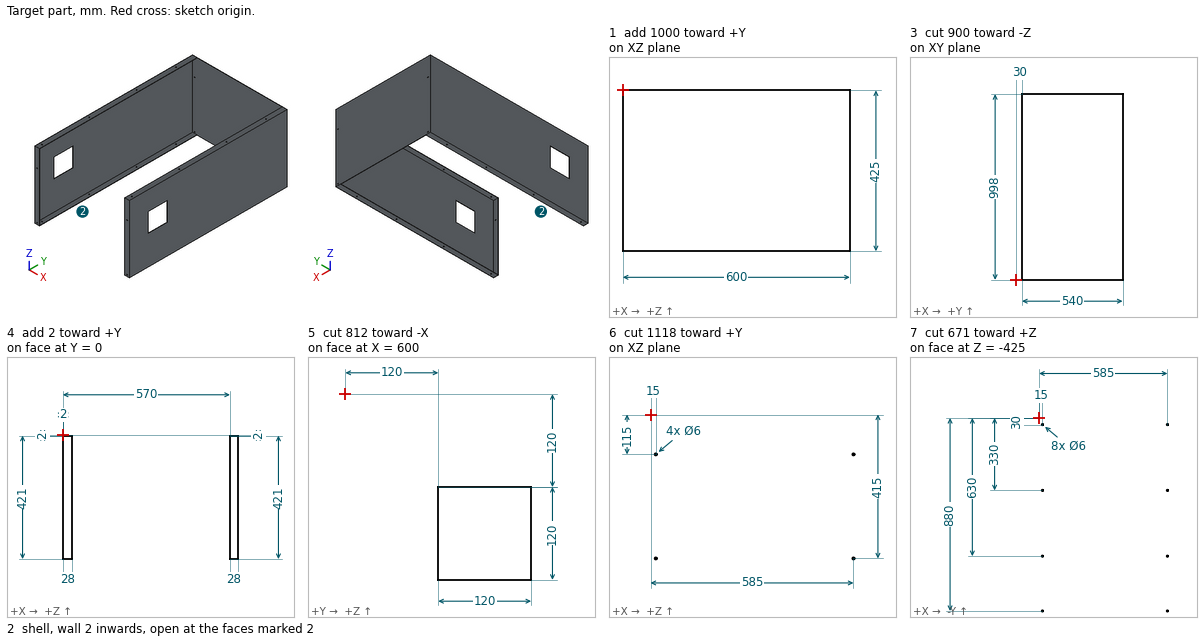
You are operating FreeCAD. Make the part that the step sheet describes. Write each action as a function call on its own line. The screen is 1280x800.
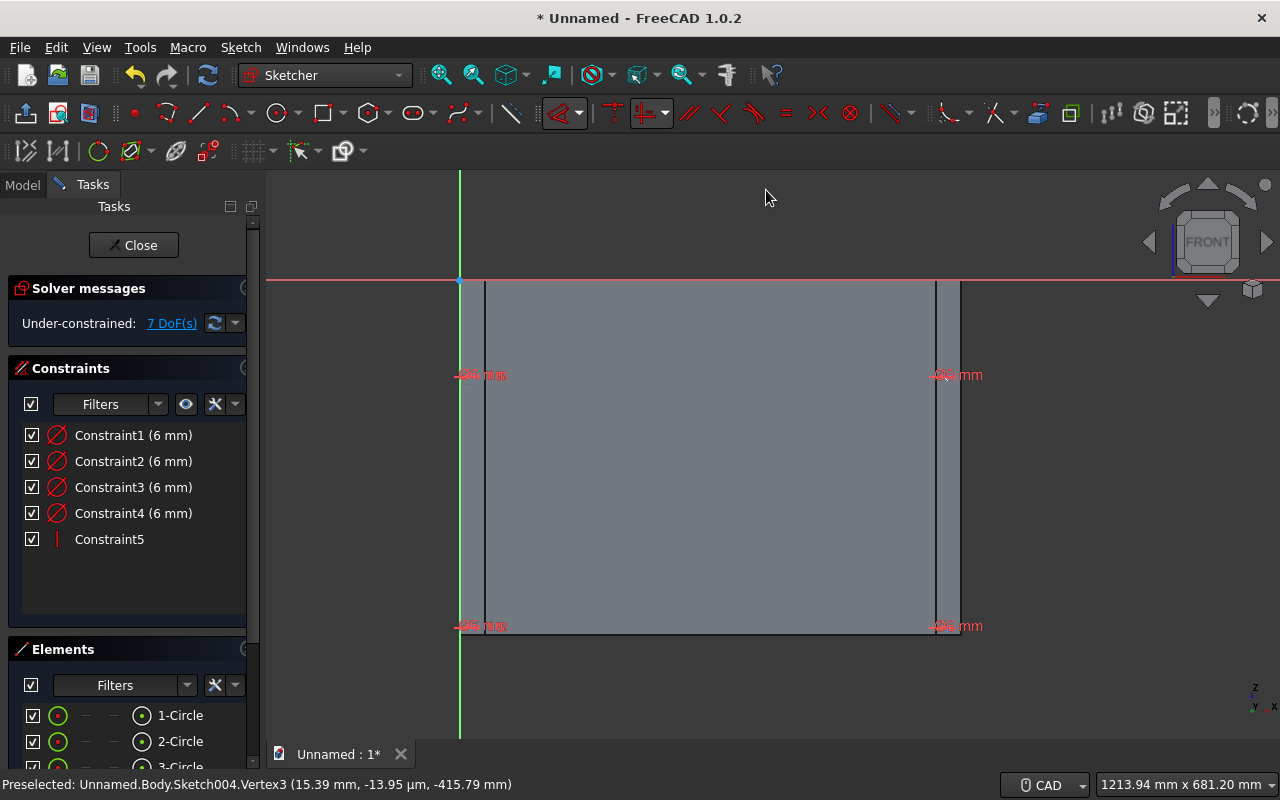
click(948, 628)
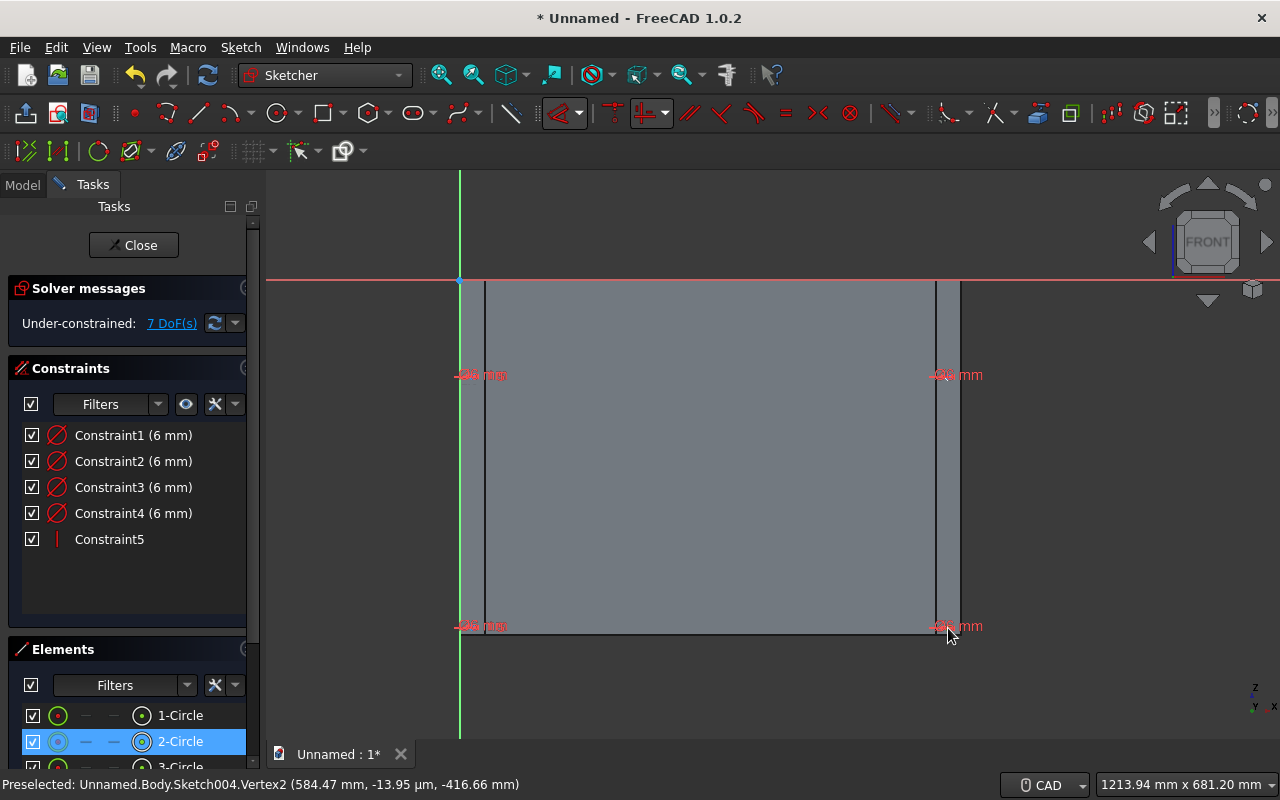
click(472, 628)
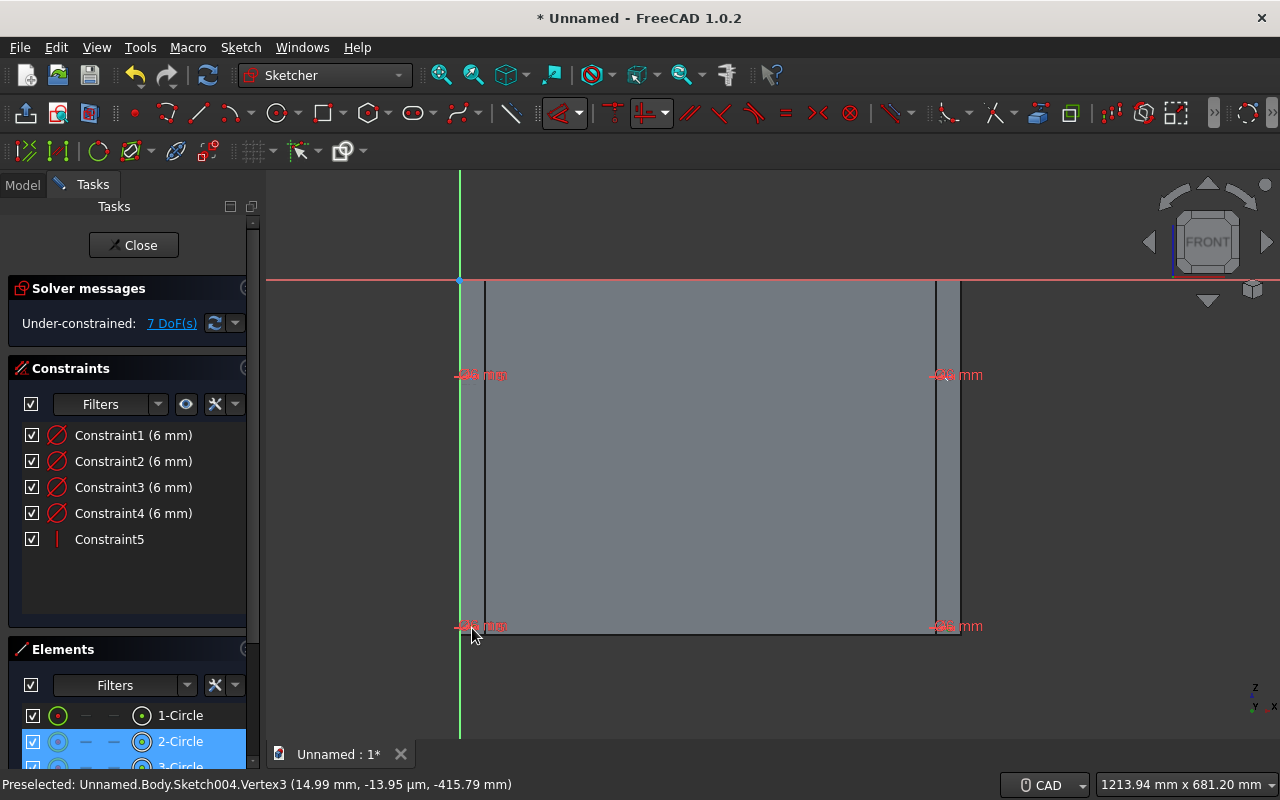
click(668, 114)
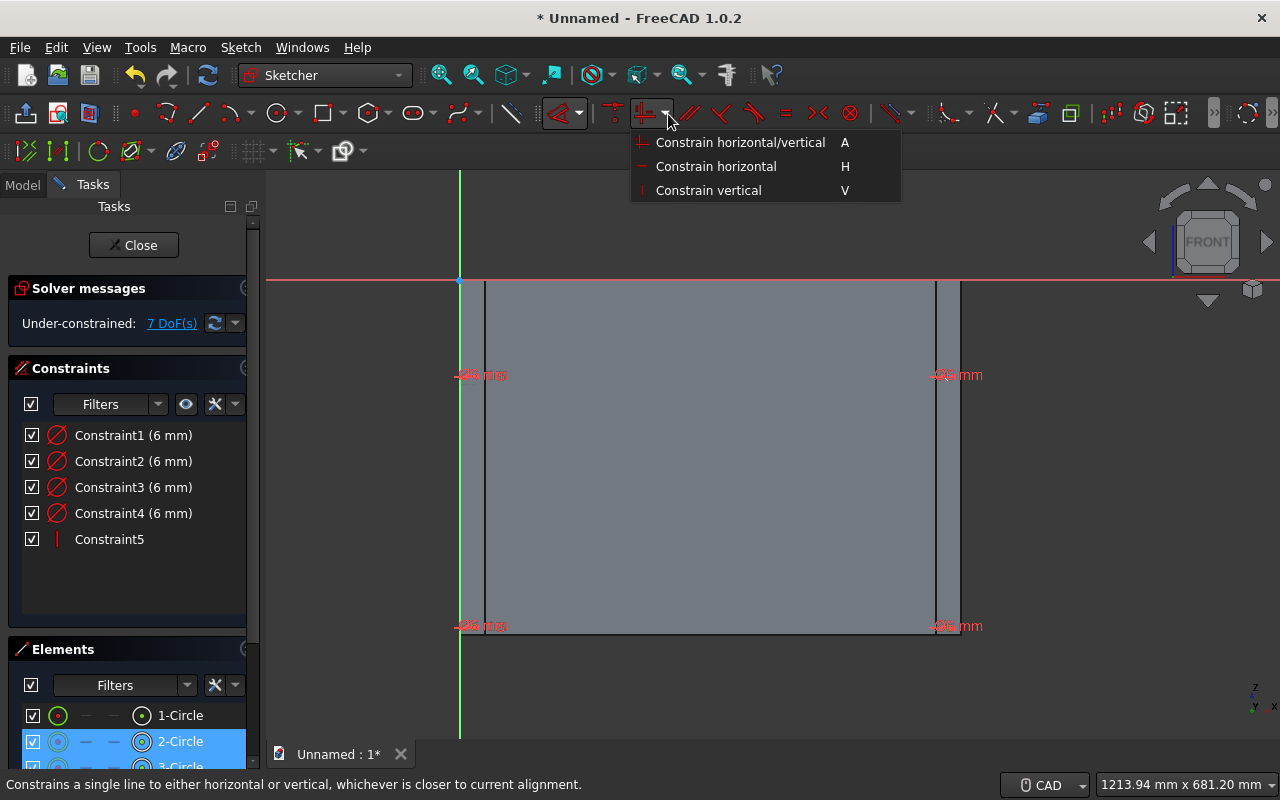
click(766, 166)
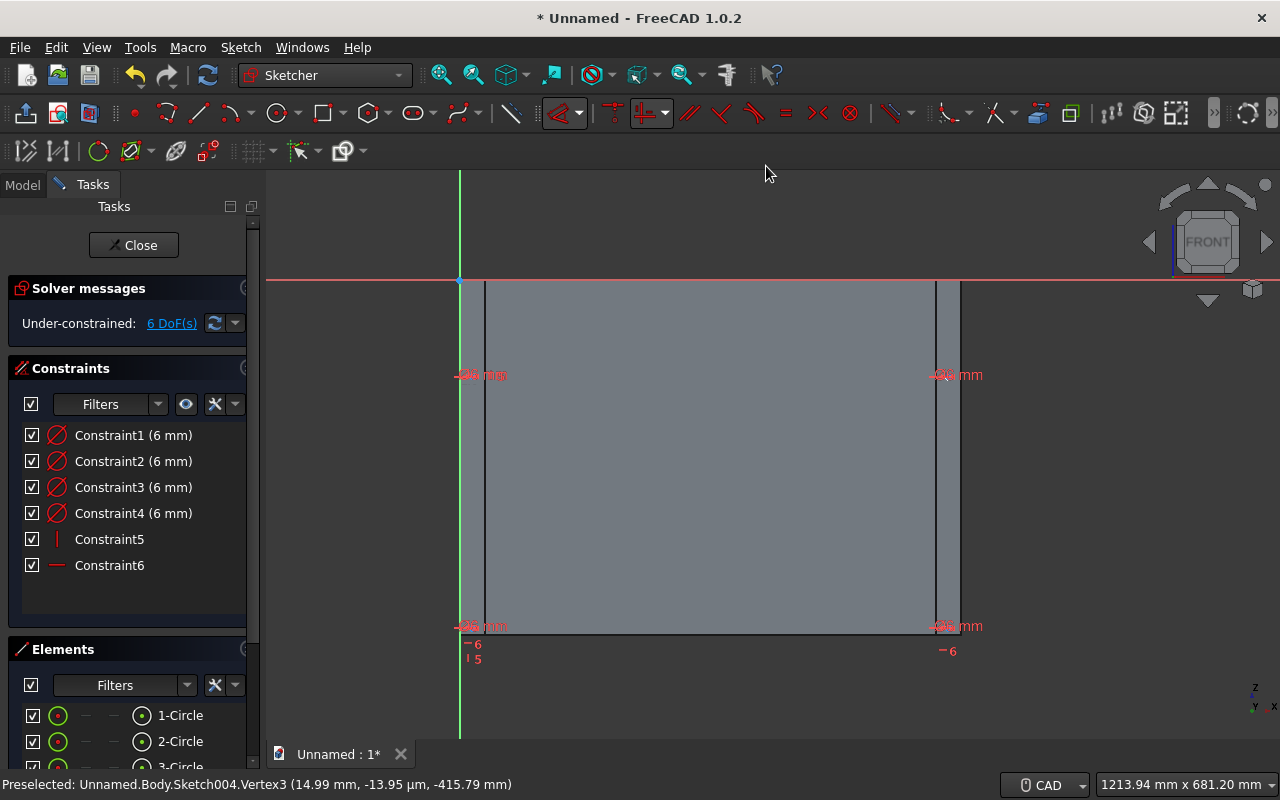
click(948, 628)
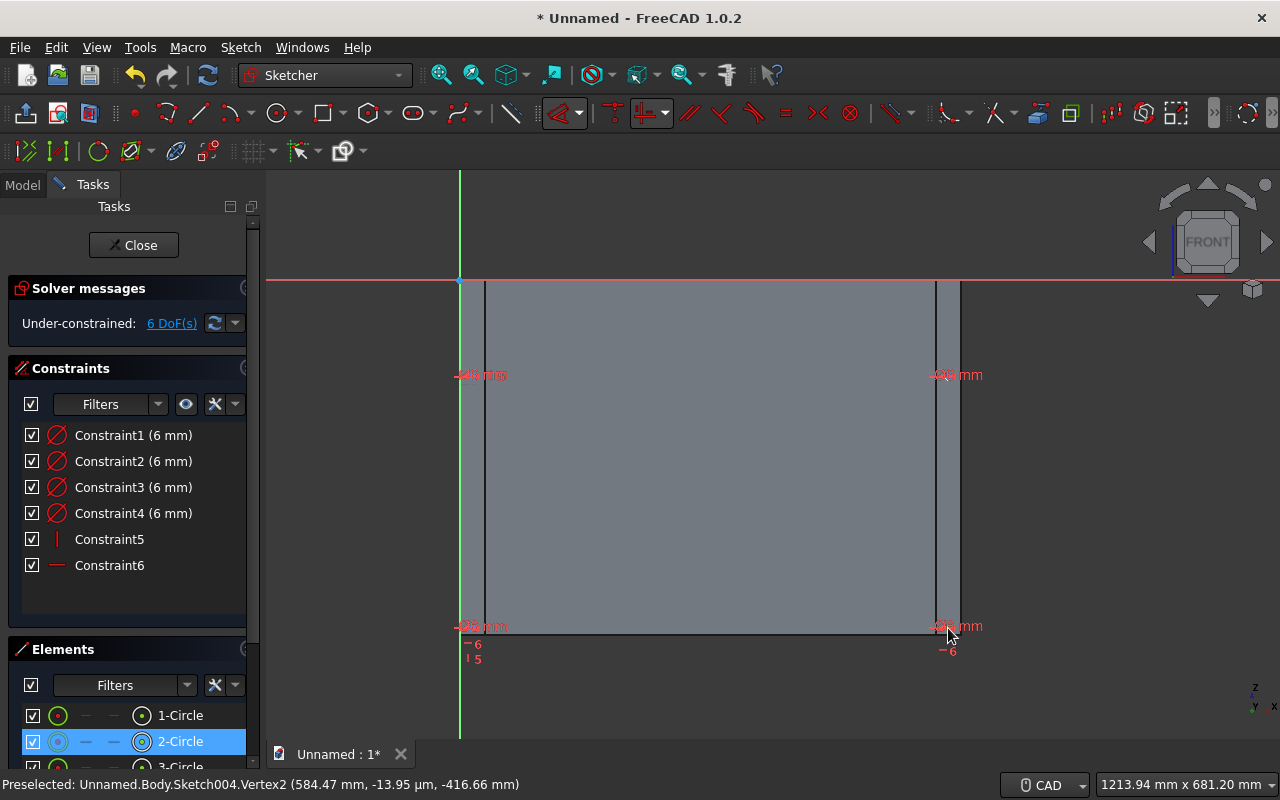
click(948, 377)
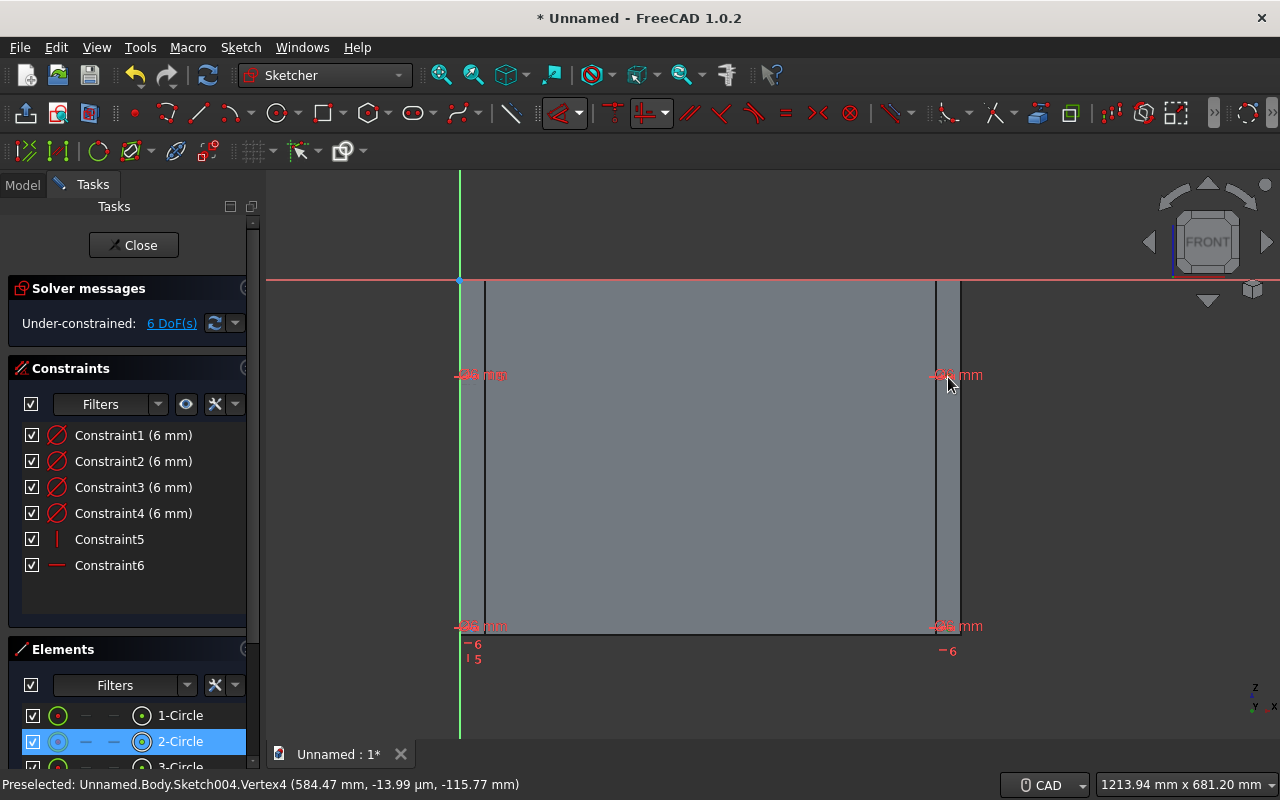
click(668, 114)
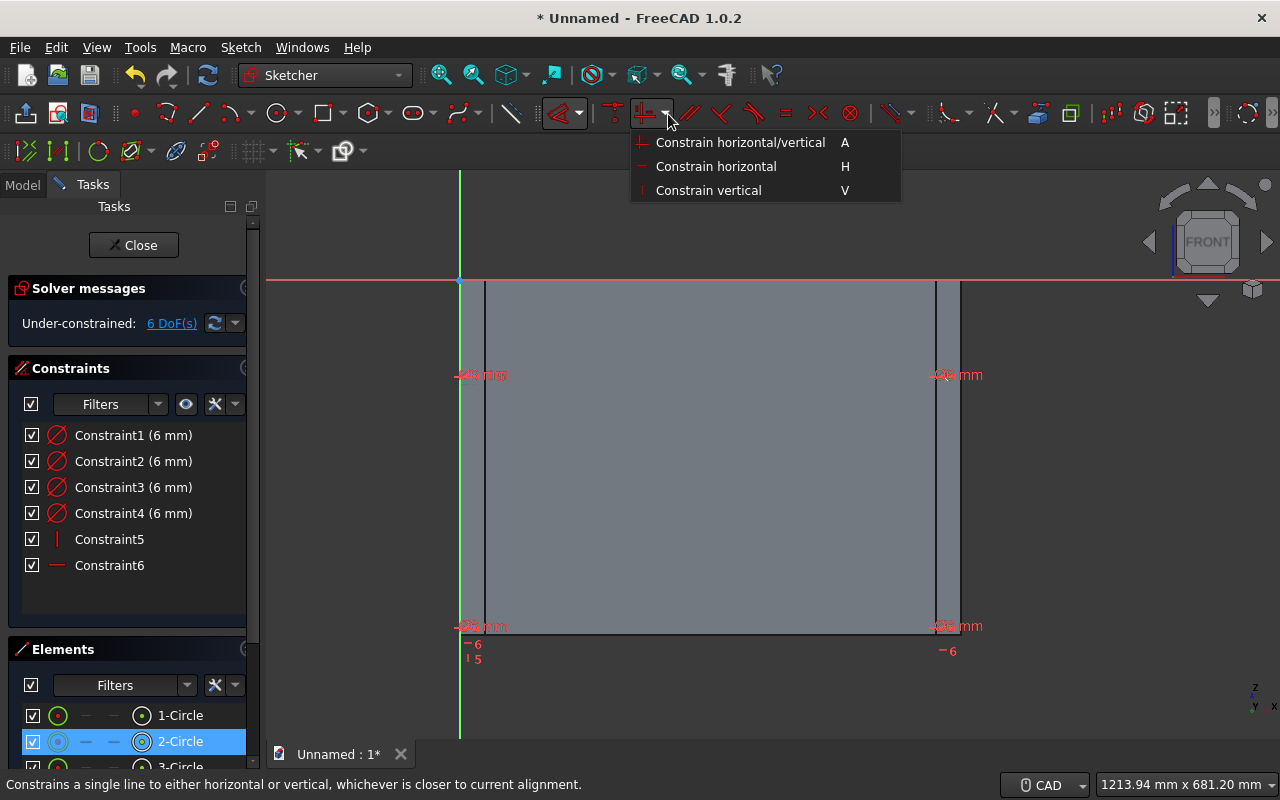
click(766, 190)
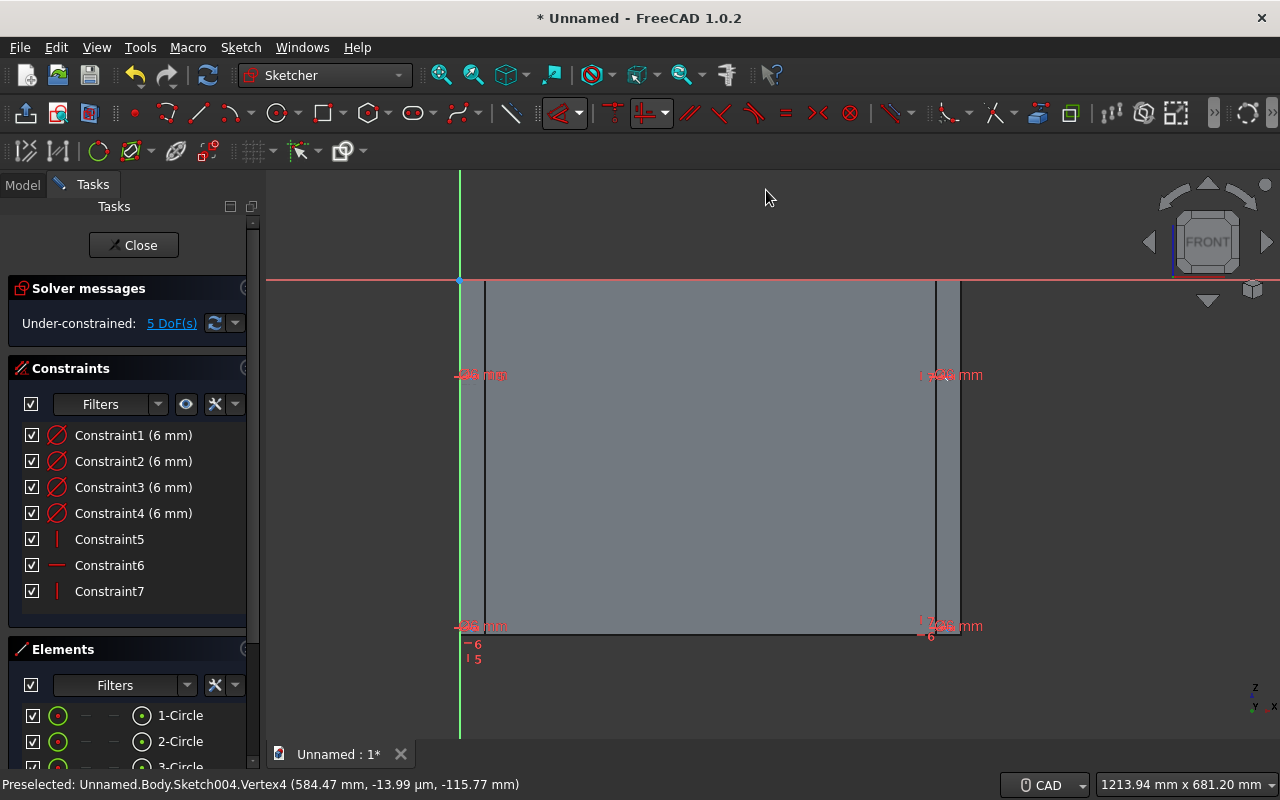
click(472, 377)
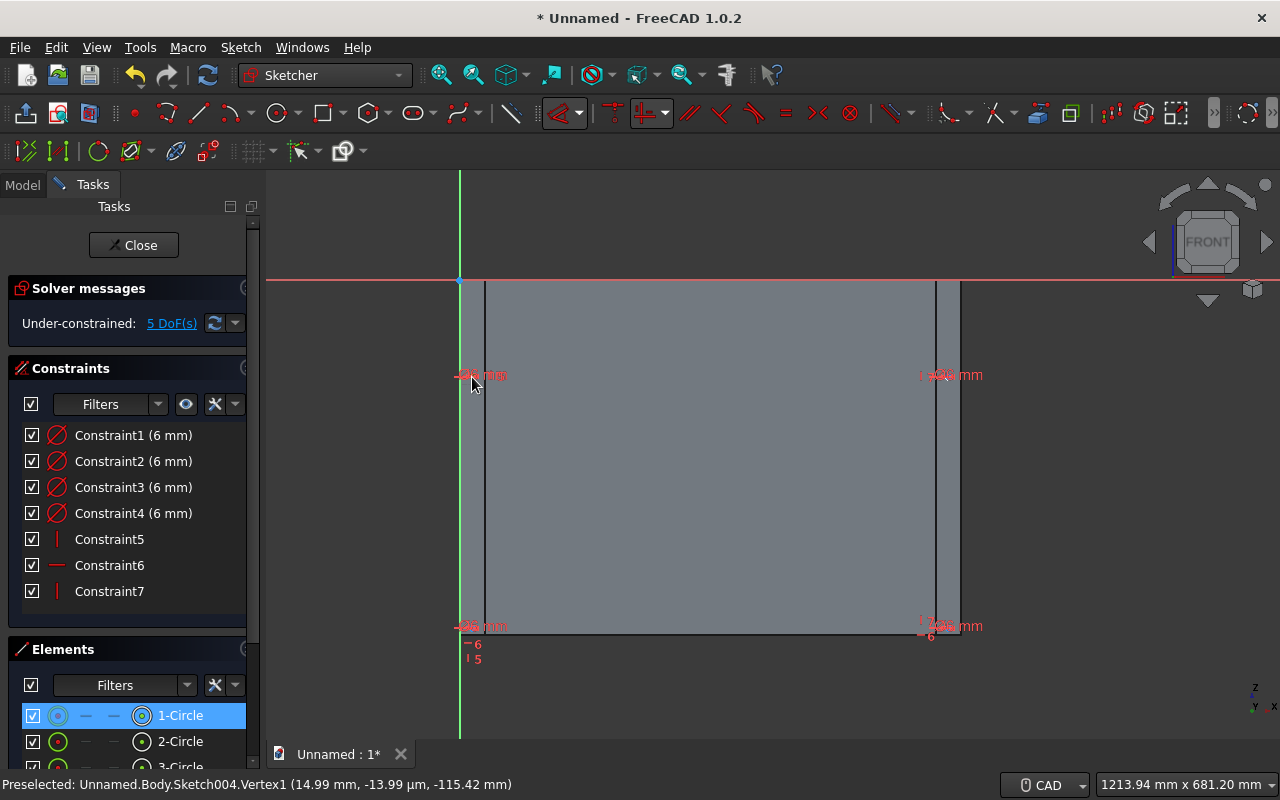
click(948, 377)